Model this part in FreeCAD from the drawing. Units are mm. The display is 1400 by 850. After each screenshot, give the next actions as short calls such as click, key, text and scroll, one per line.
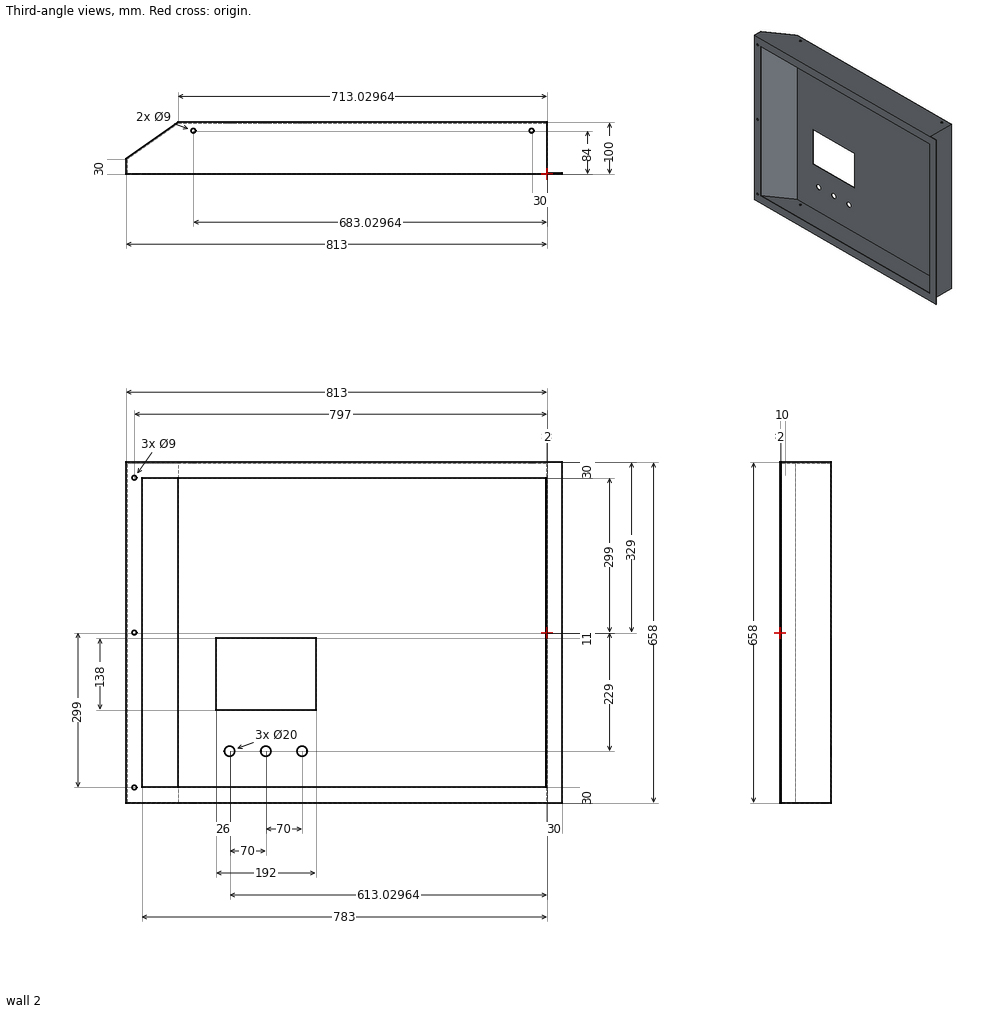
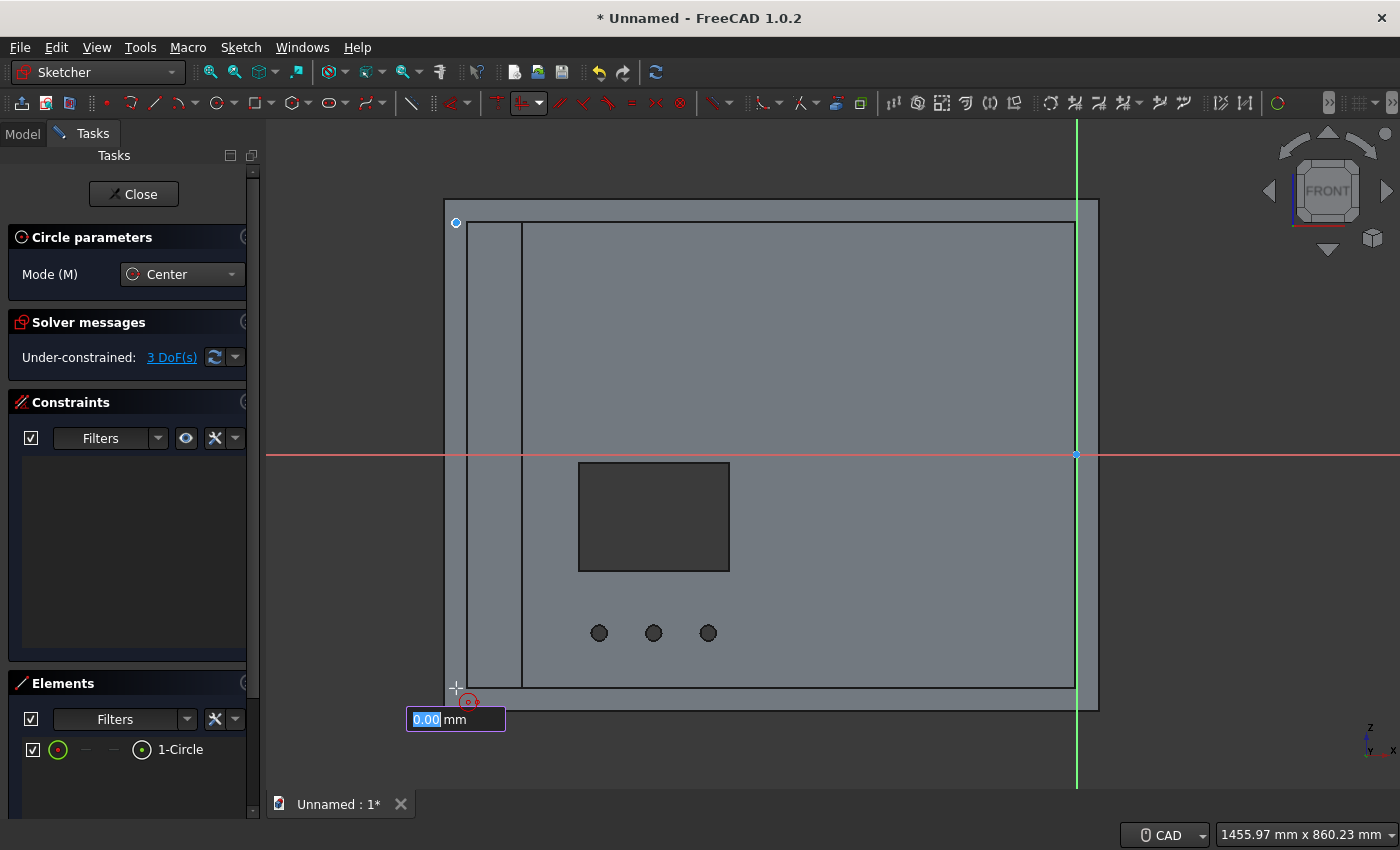
scroll(458, 685, up, 8)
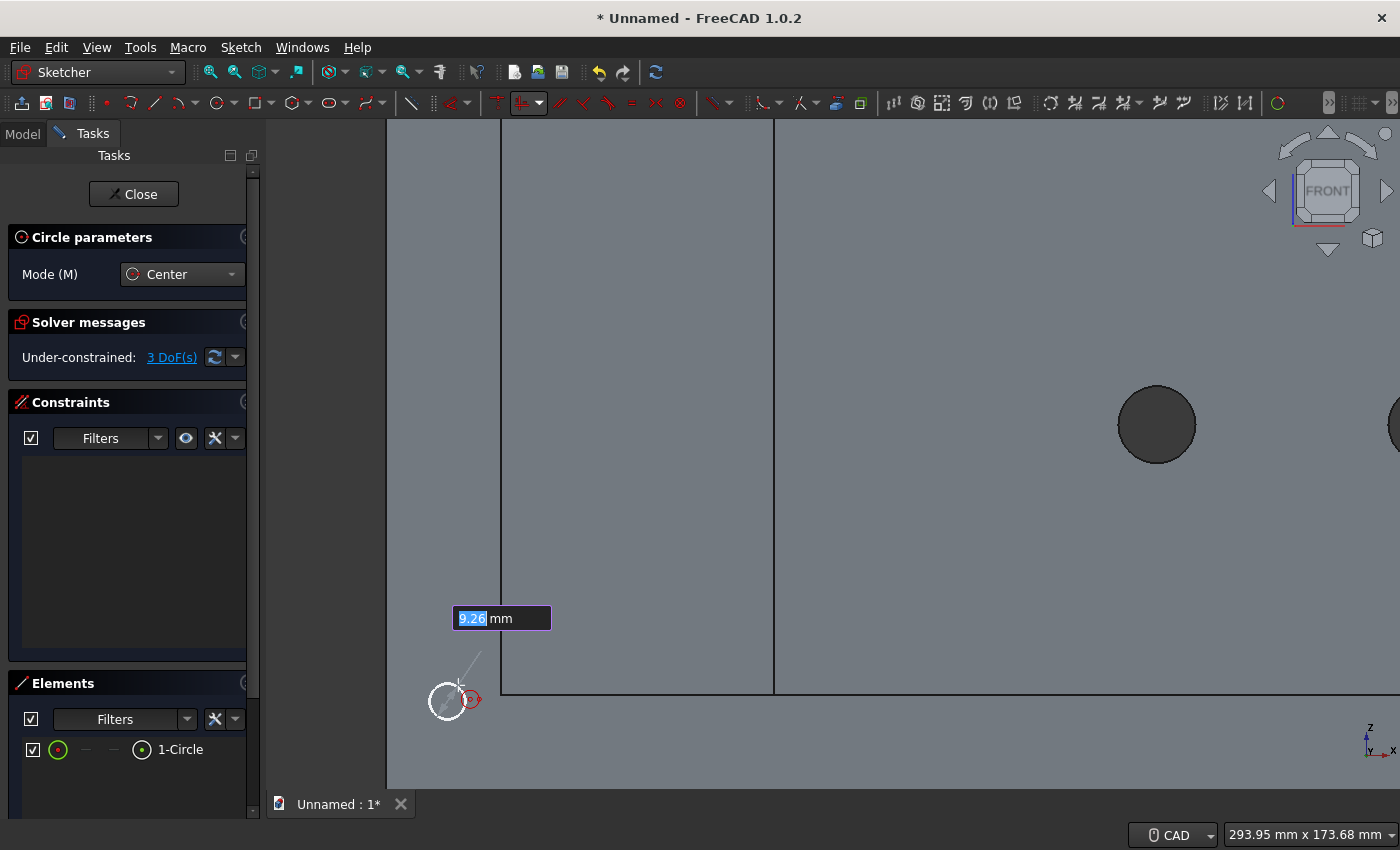
click(460, 682)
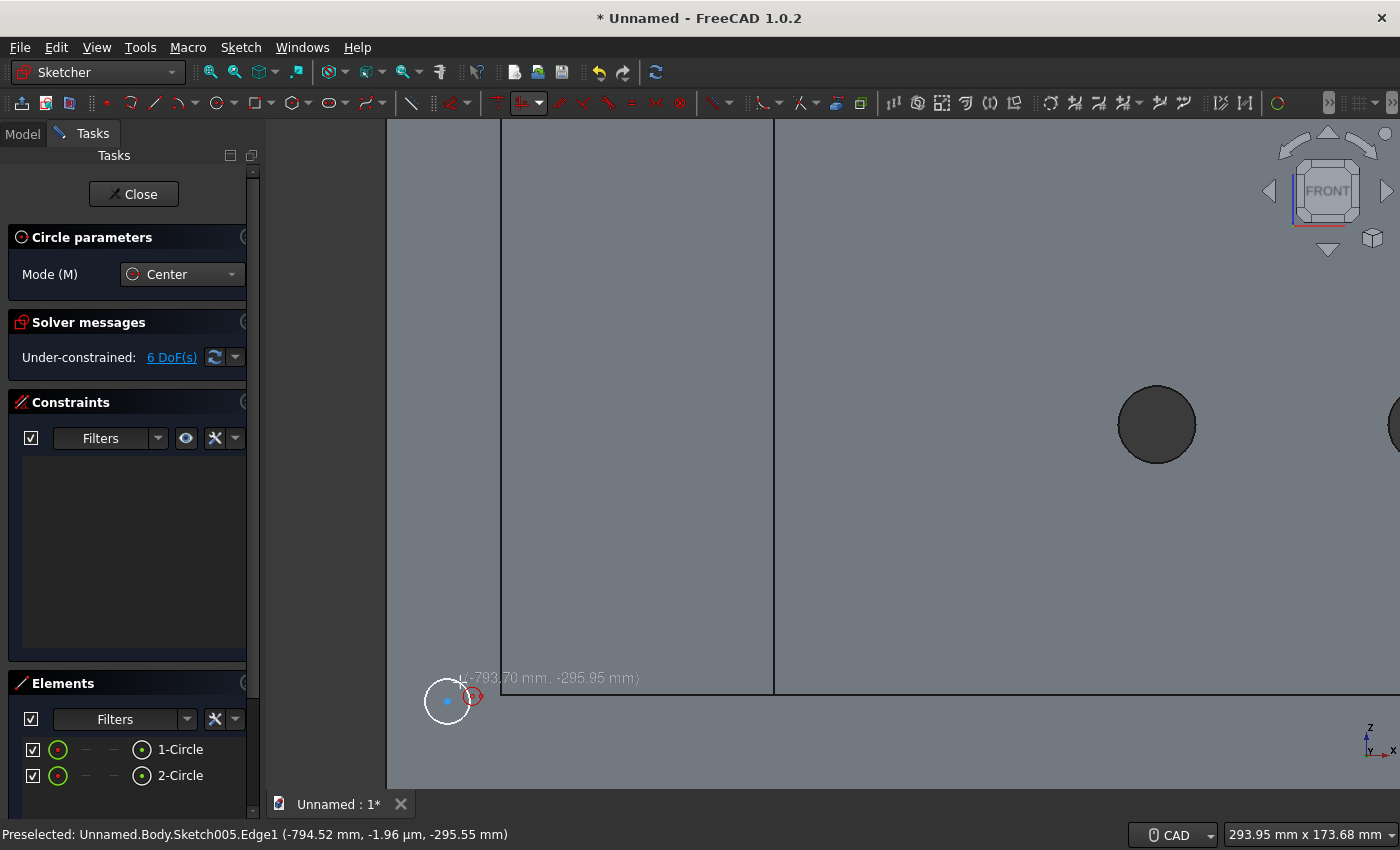
scroll(458, 685, down, 8)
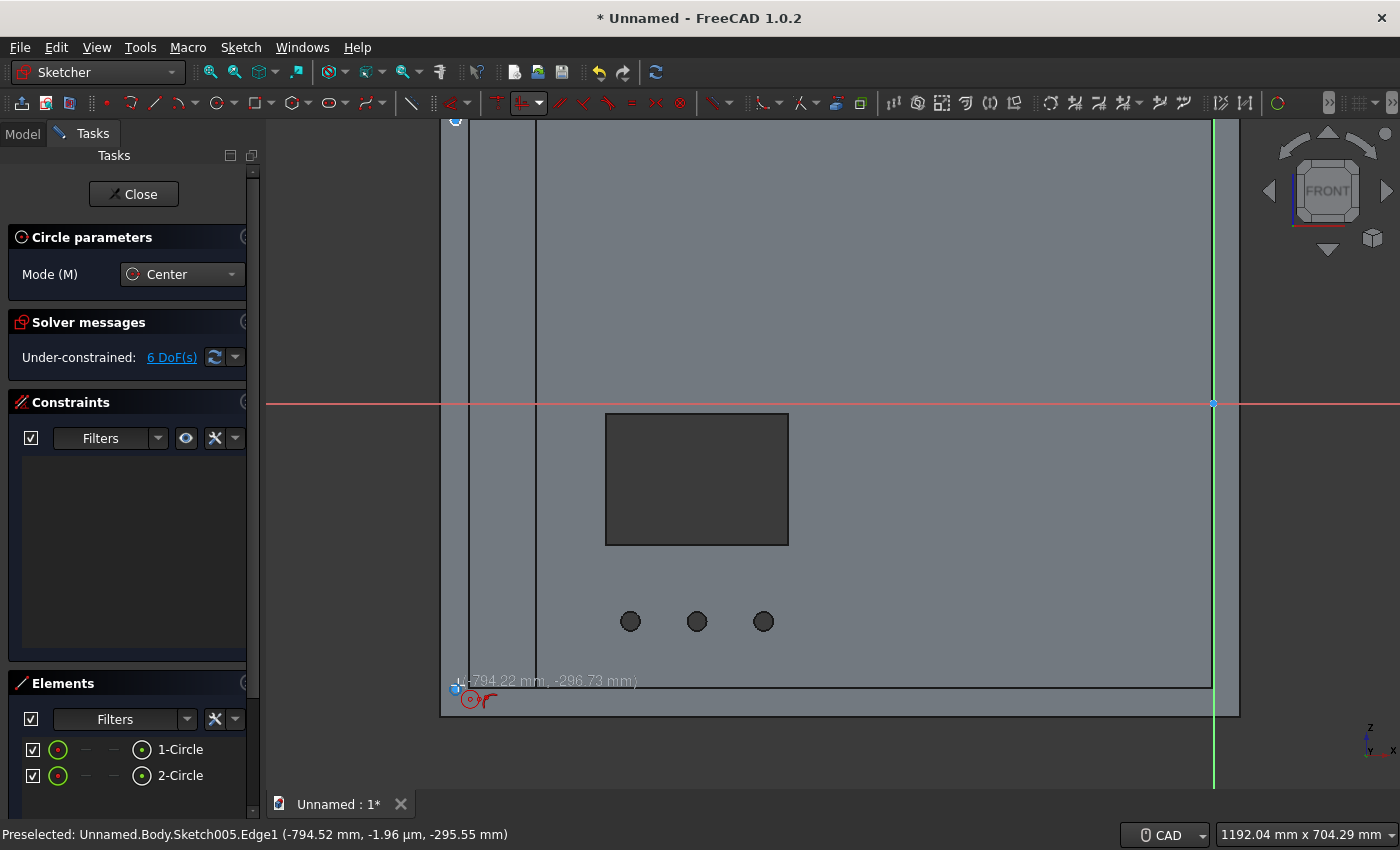
scroll(456, 455, up, 10)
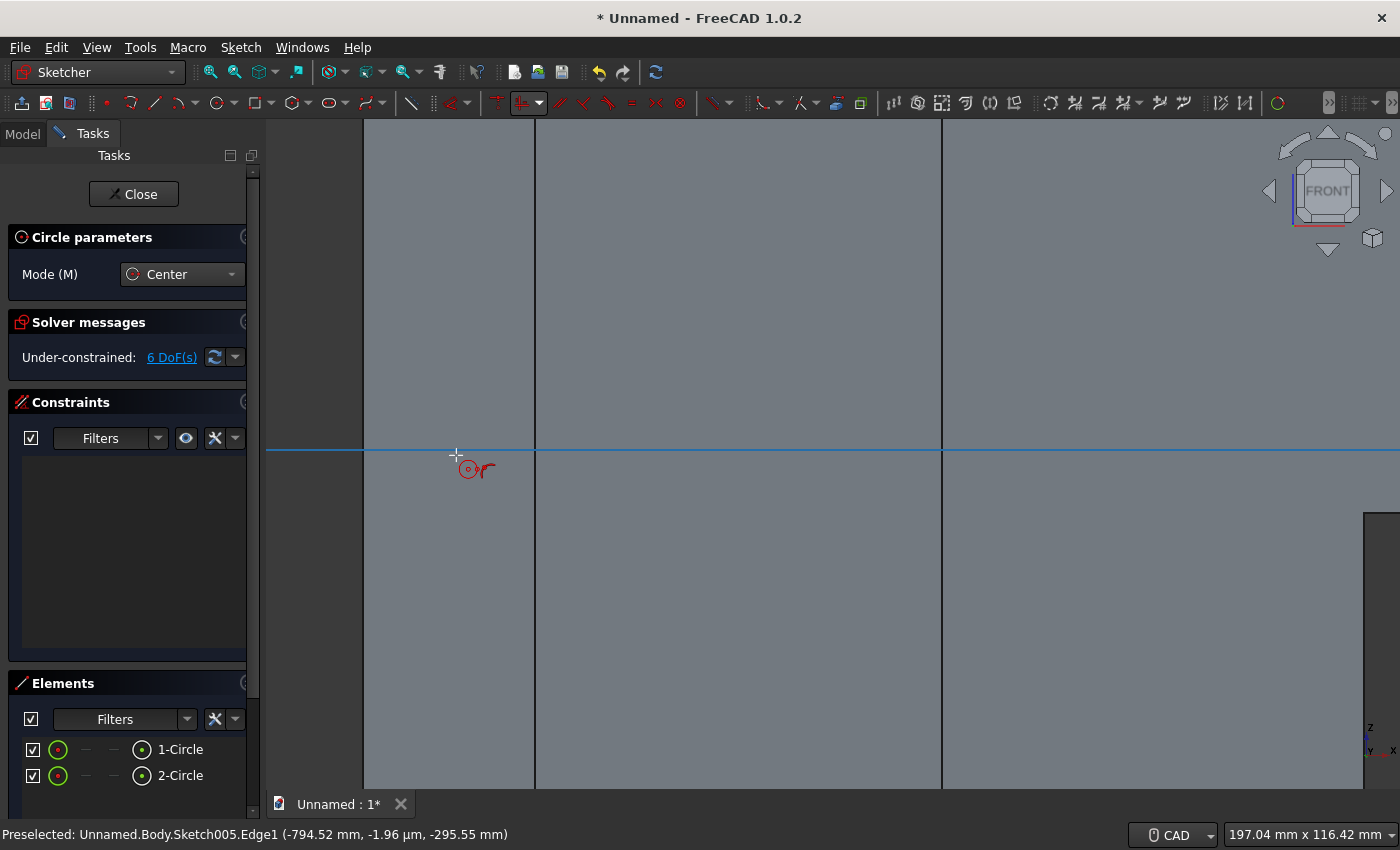
scroll(456, 455, down, 10)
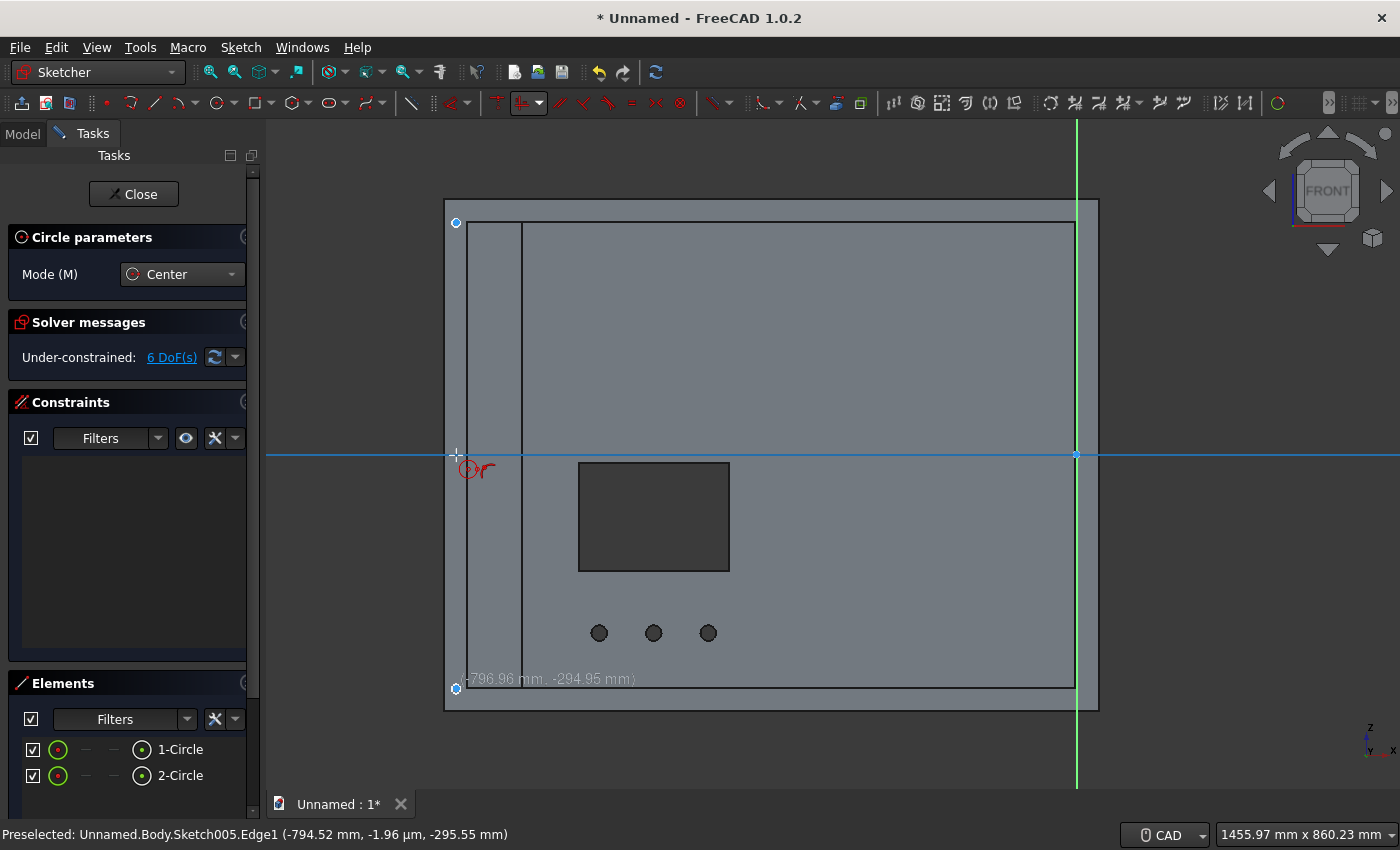
click(456, 455)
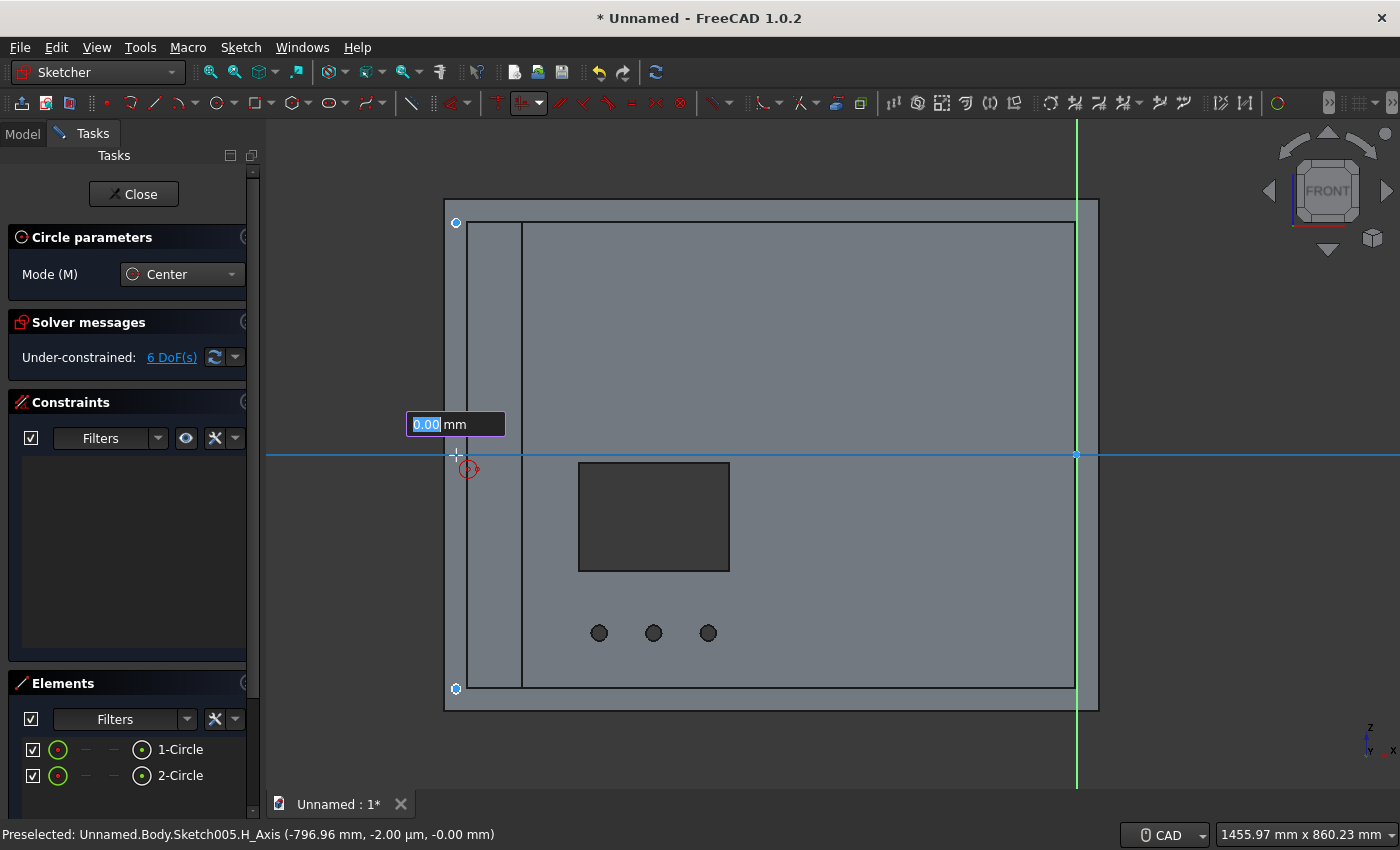
scroll(455, 458, up, 8)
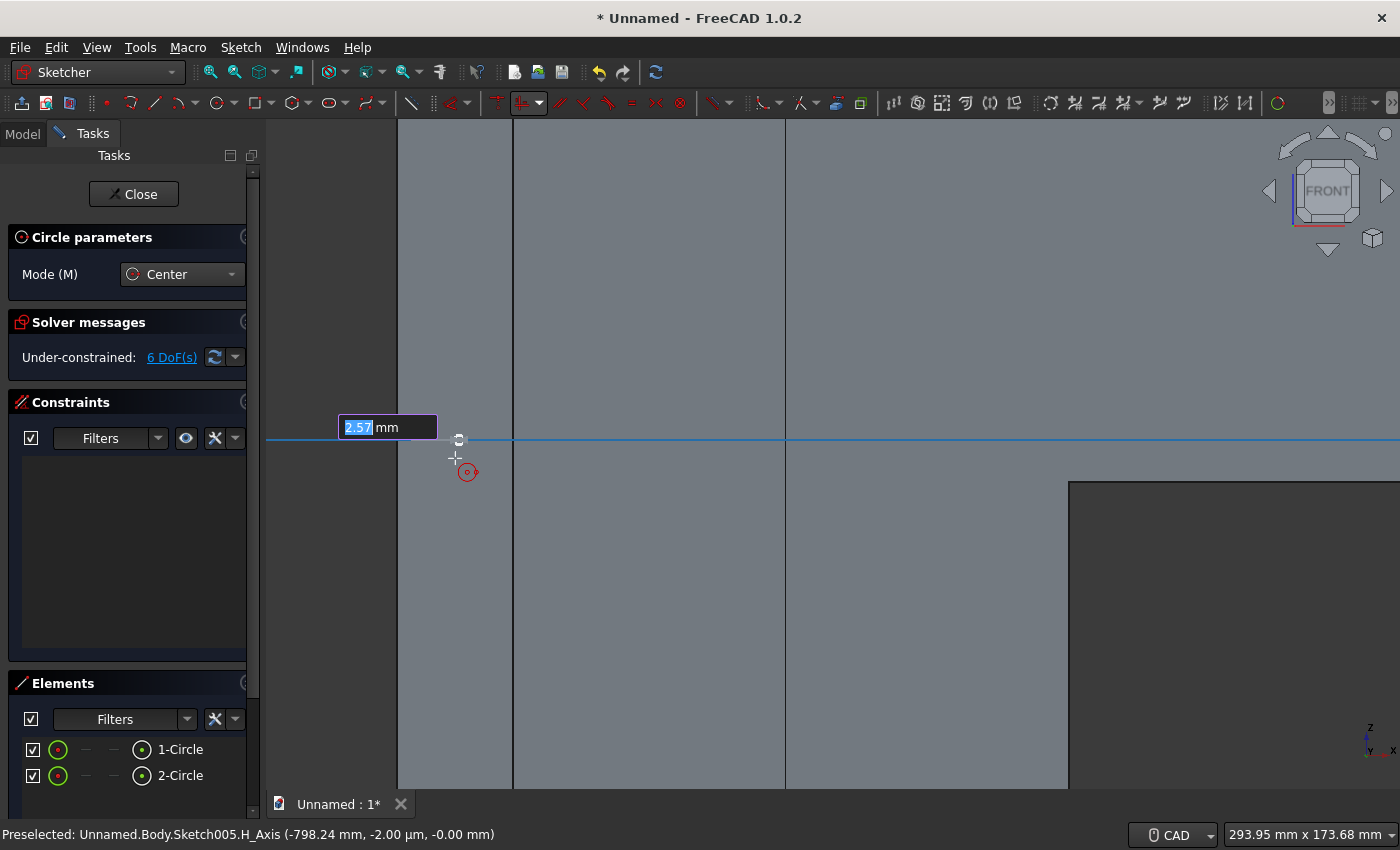
click(453, 456)
key(Escape)